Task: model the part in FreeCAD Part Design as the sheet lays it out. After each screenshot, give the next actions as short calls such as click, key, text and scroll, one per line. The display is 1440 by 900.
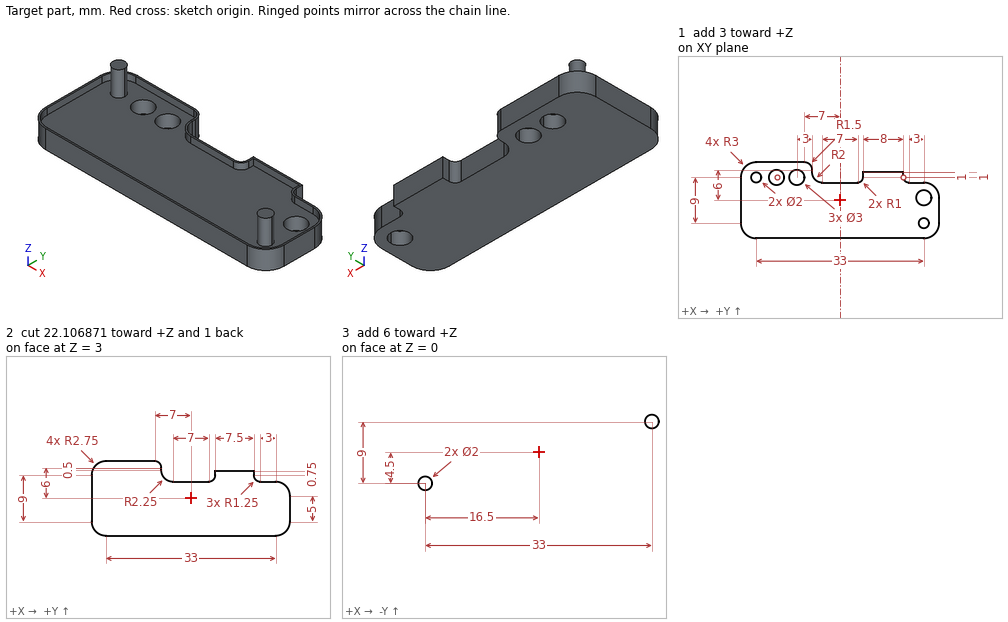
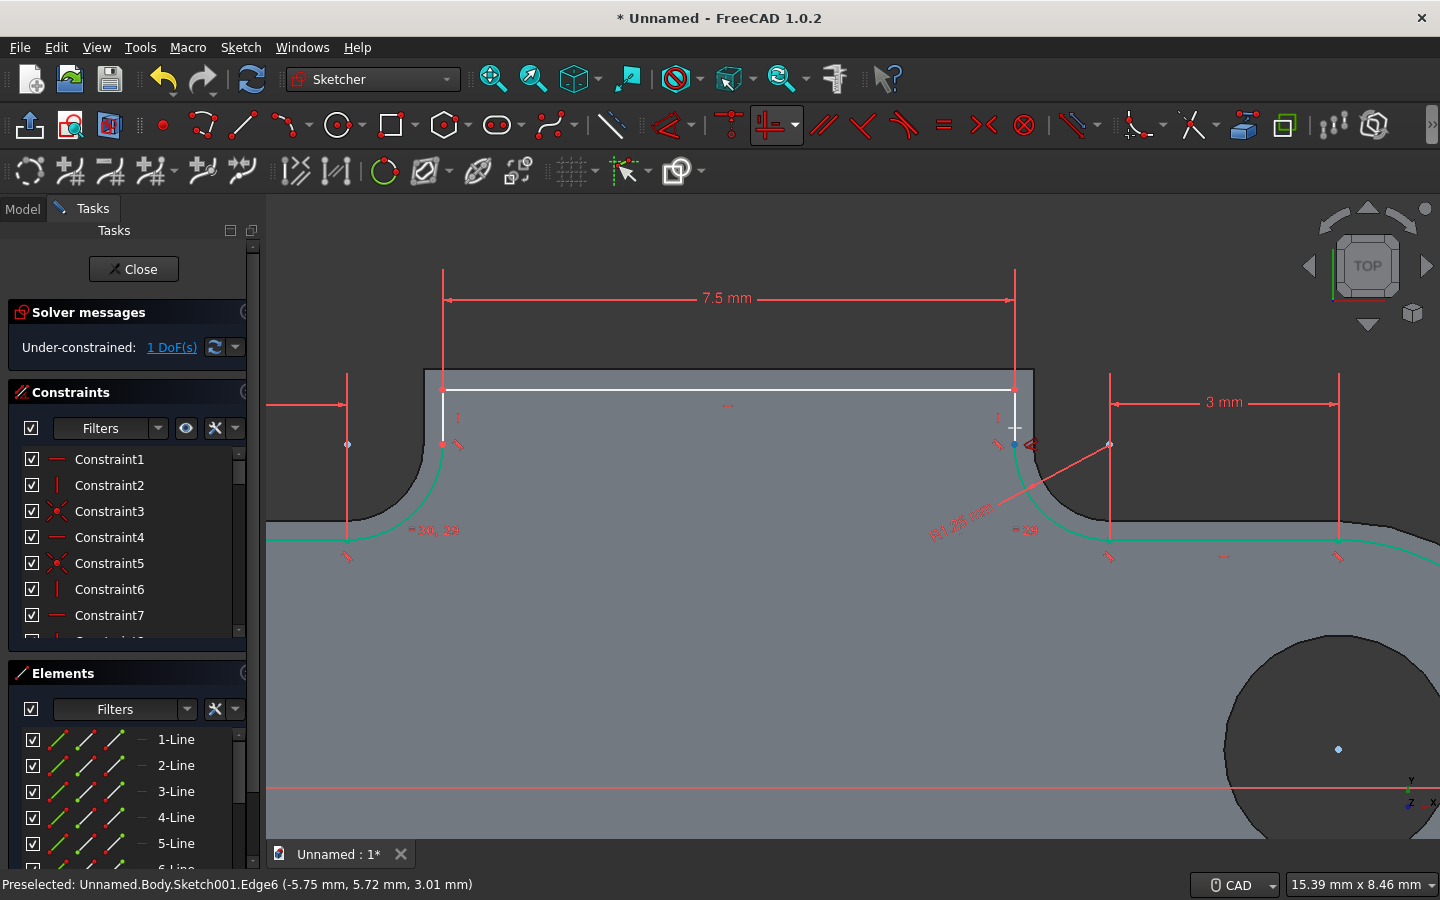
click(1015, 428)
click(1049, 417)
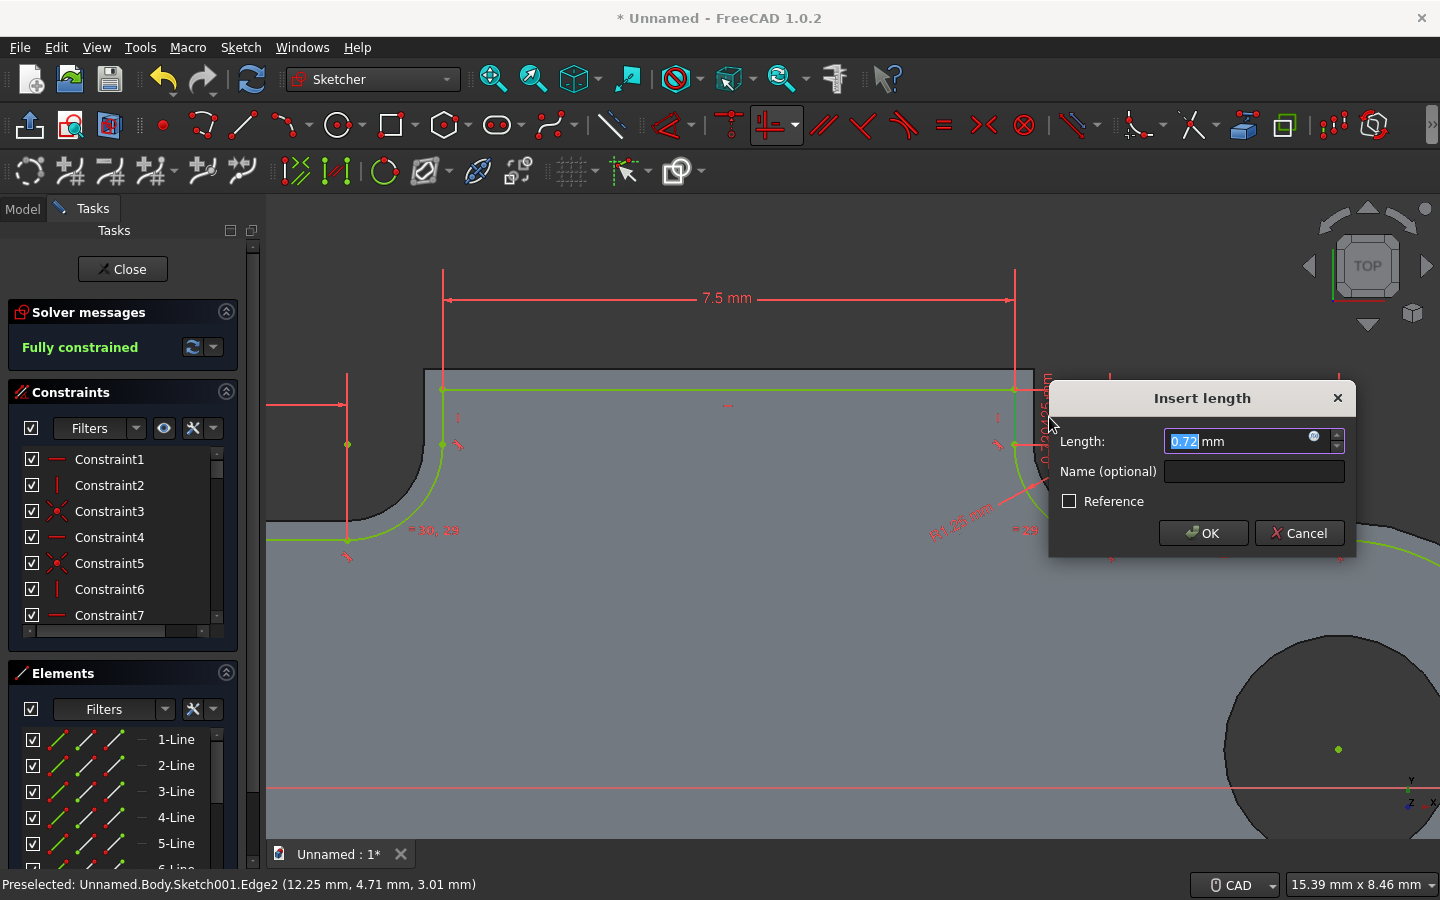
text(0.75)
key(Return)
key(Escape)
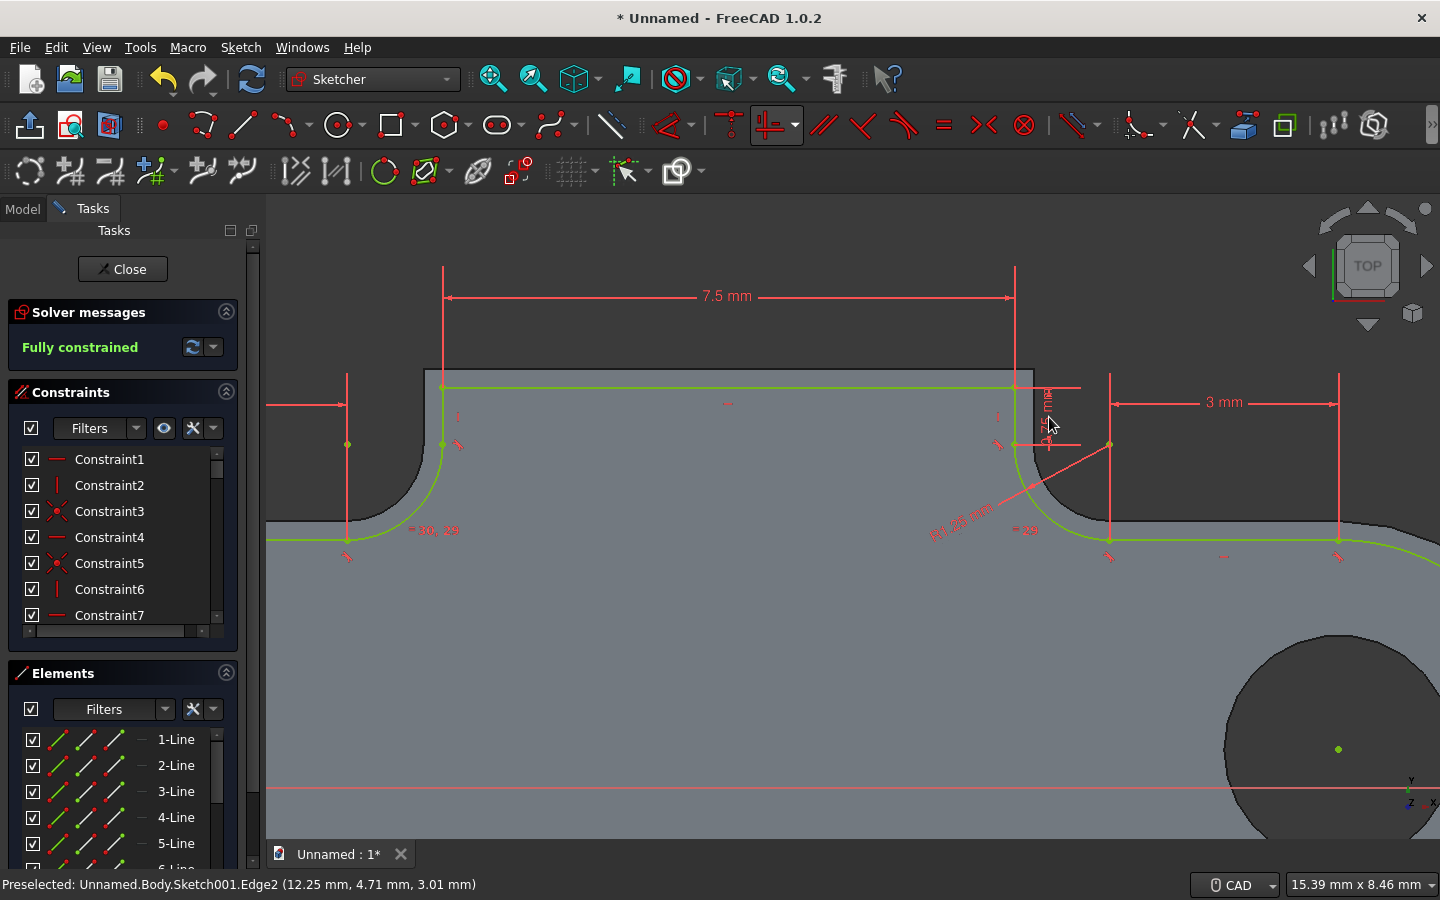
click(123, 269)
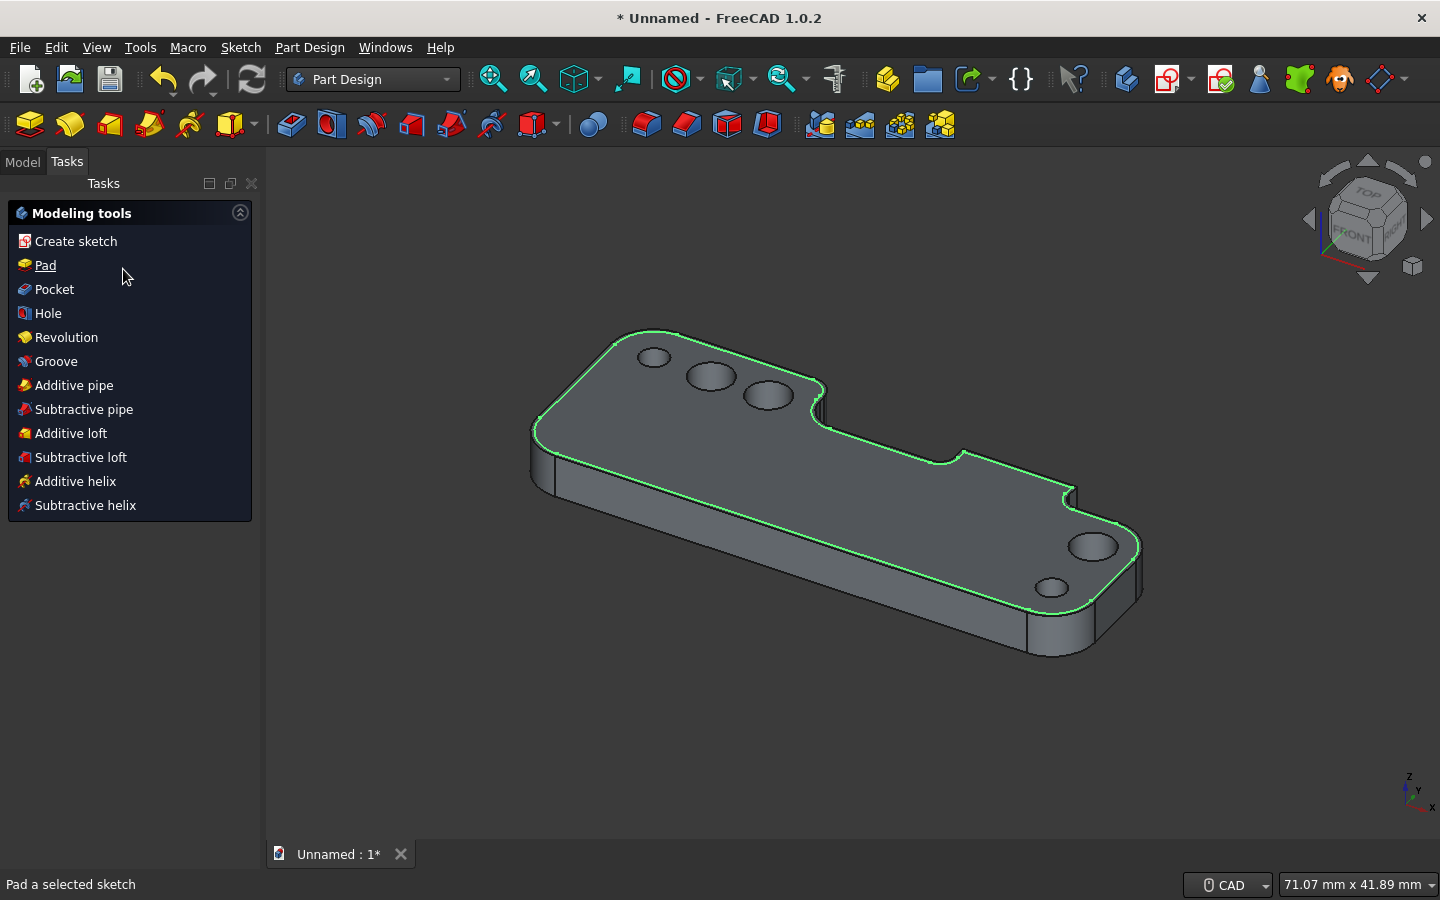
click(292, 124)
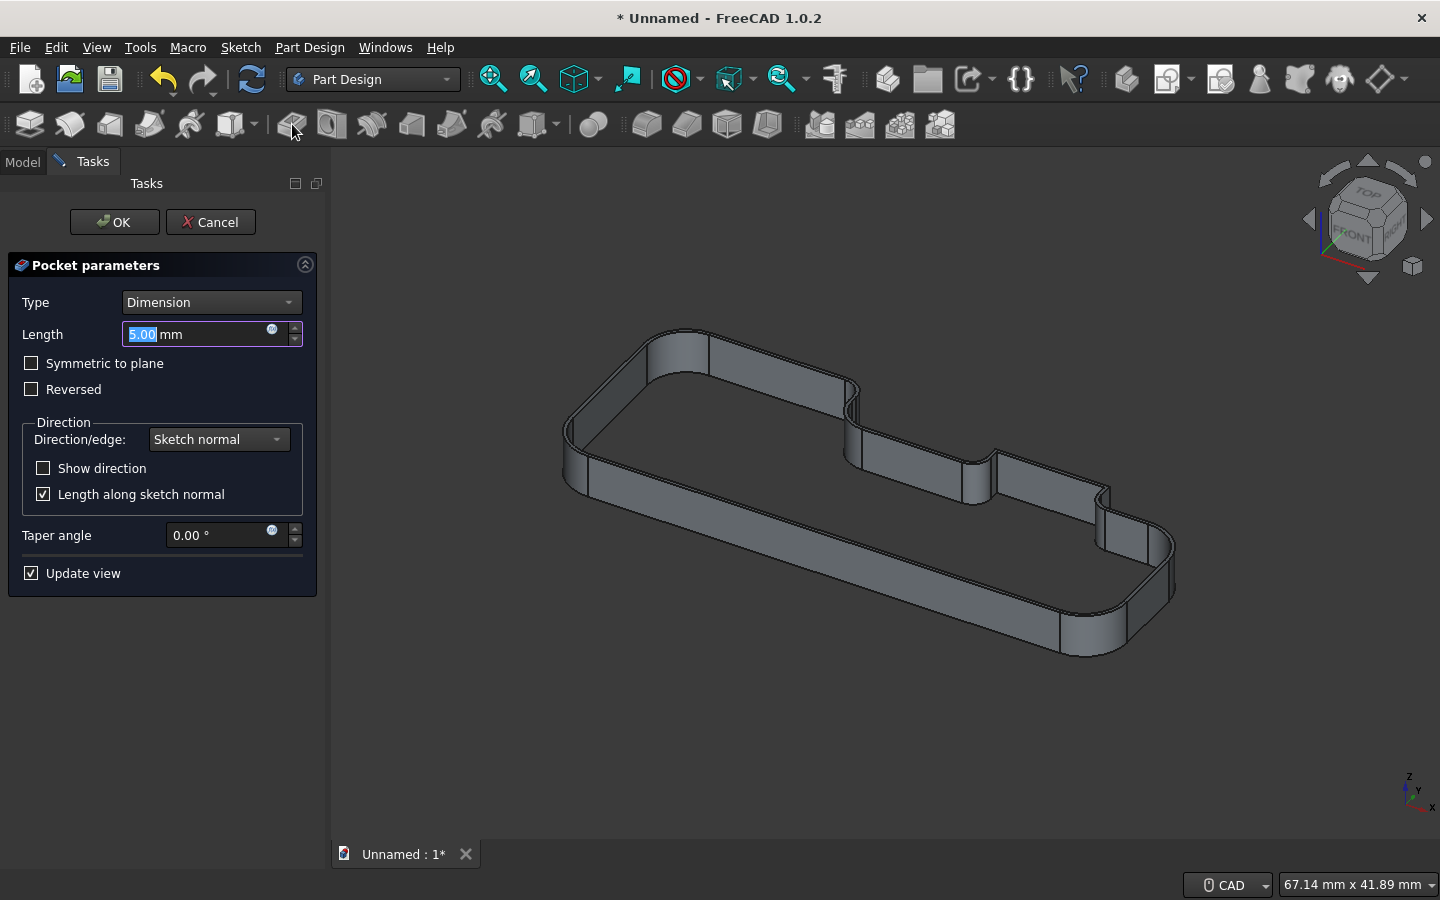
click(212, 302)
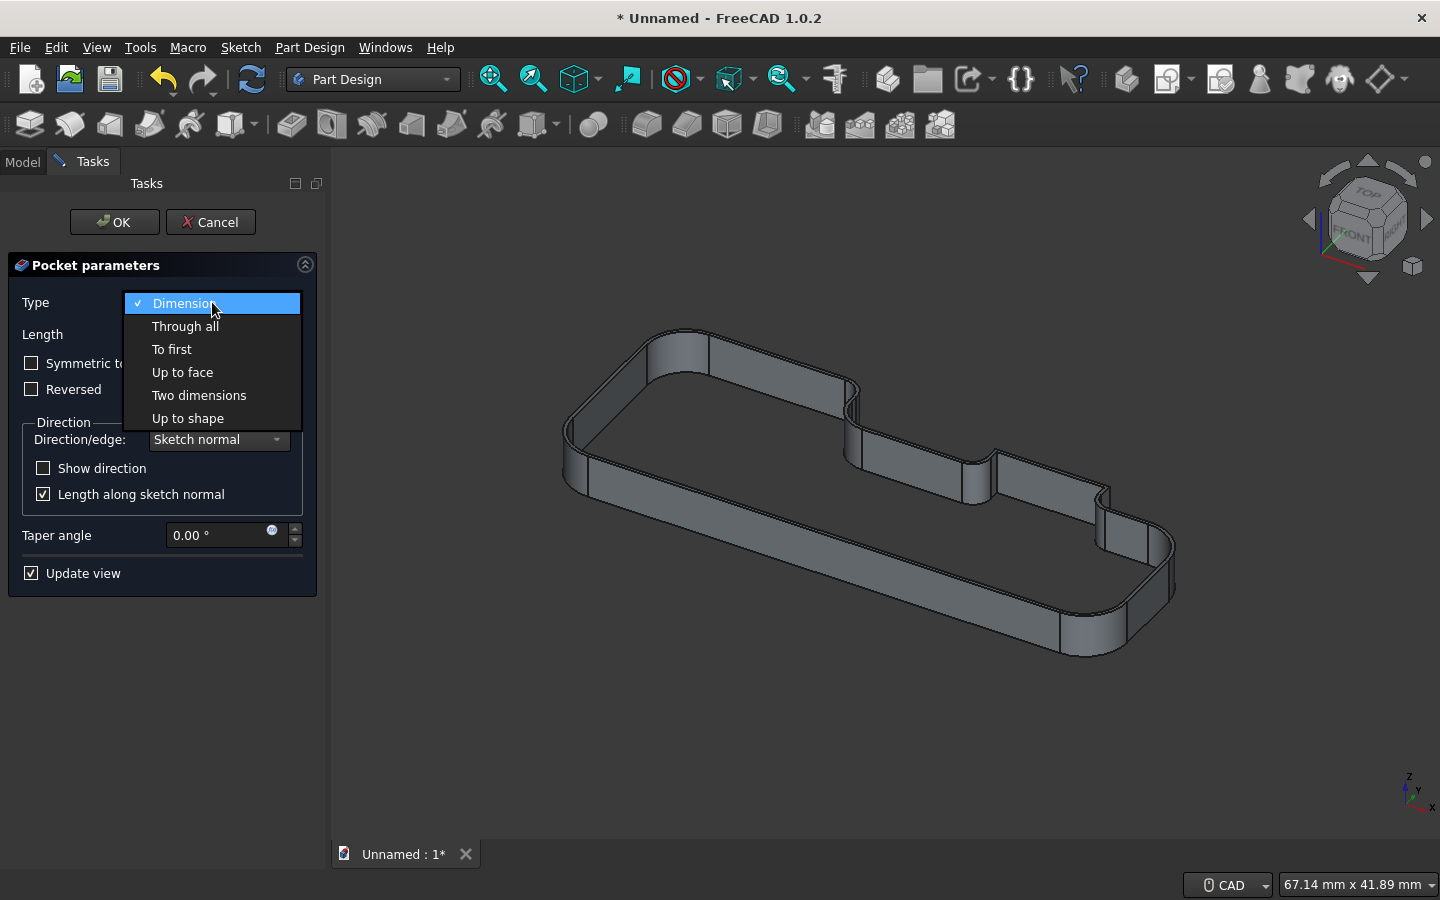
click(212, 396)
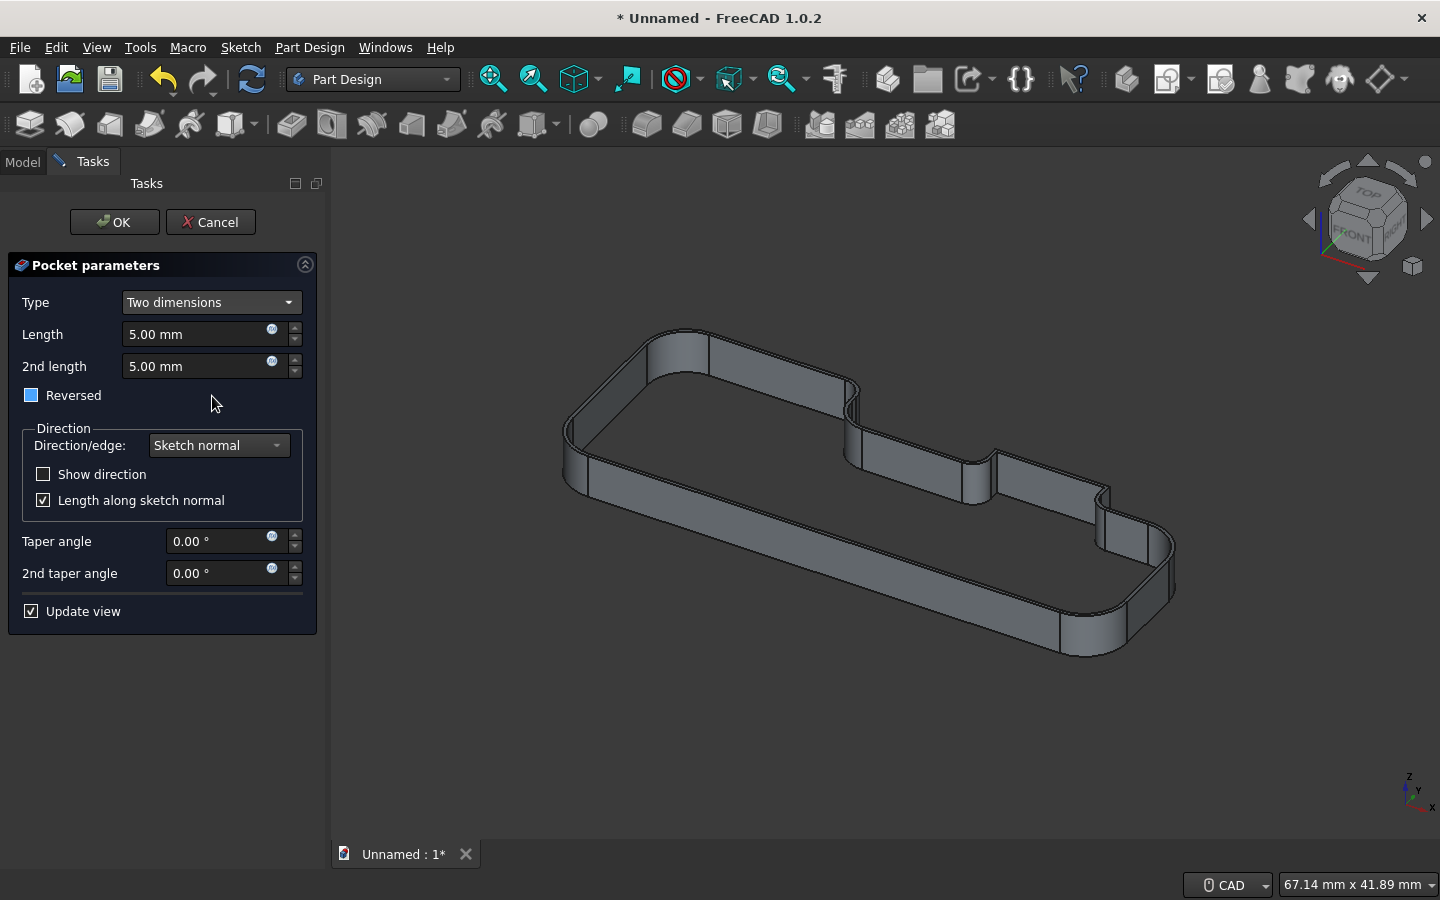
triple_click(204, 334)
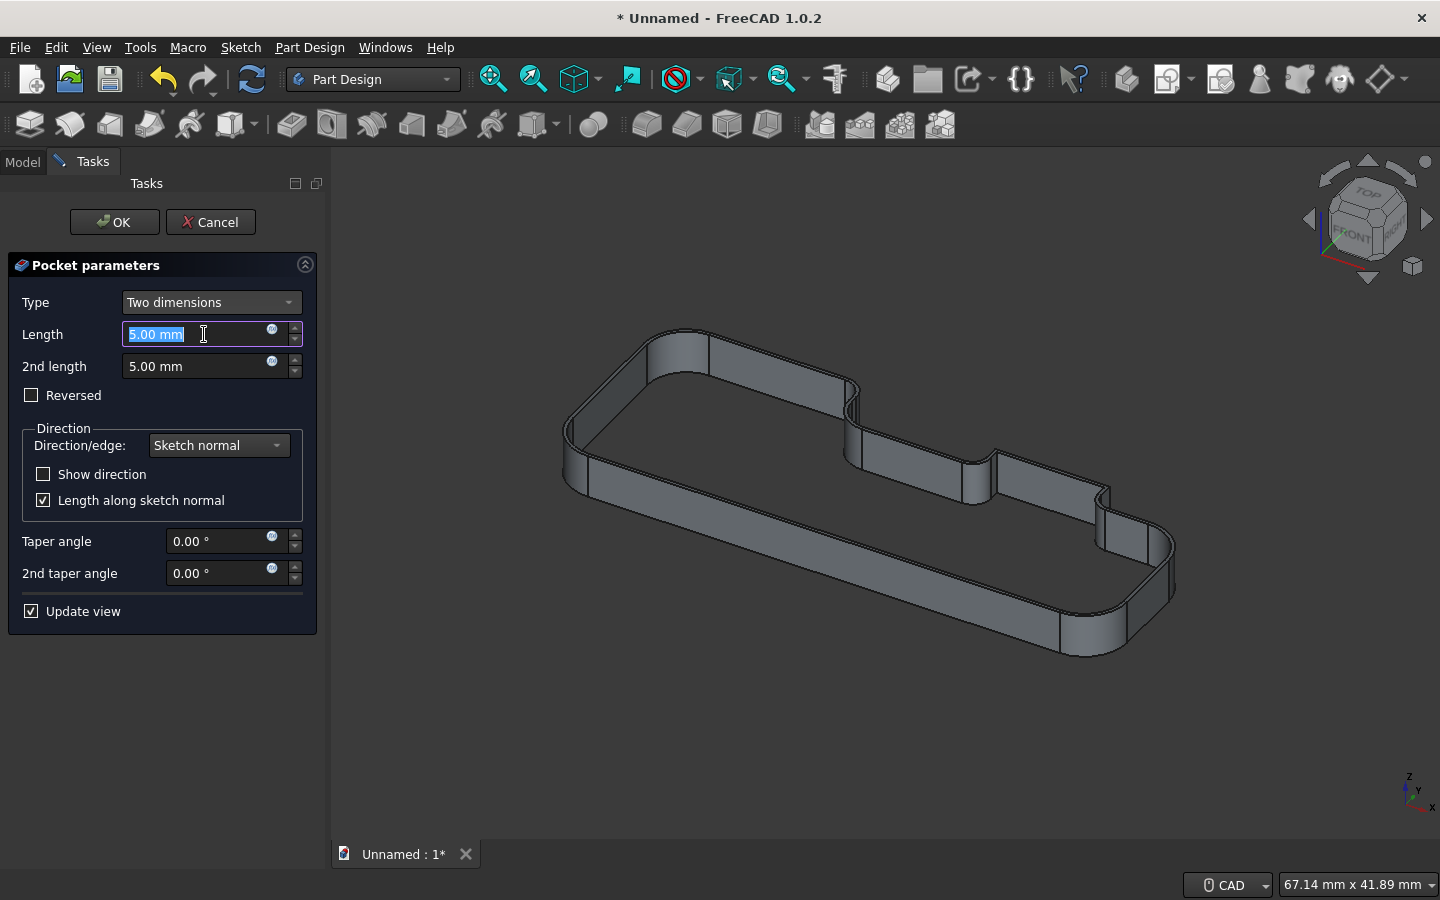
text(22.106871)
key(Tab)